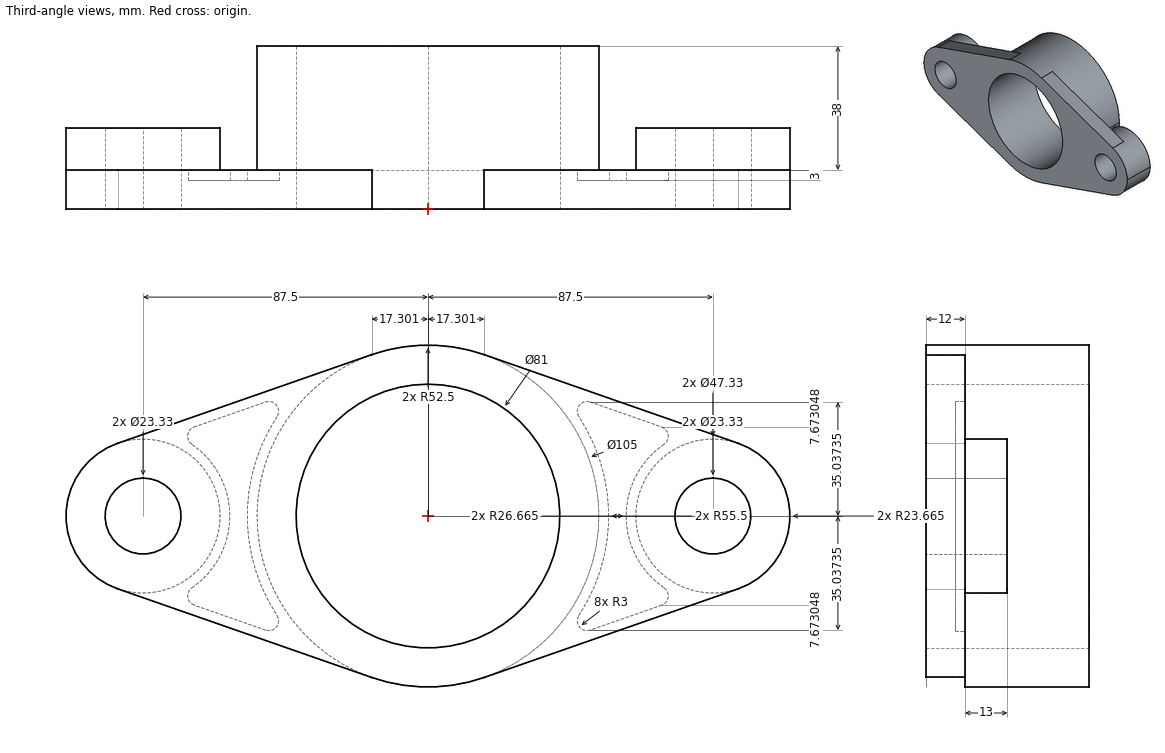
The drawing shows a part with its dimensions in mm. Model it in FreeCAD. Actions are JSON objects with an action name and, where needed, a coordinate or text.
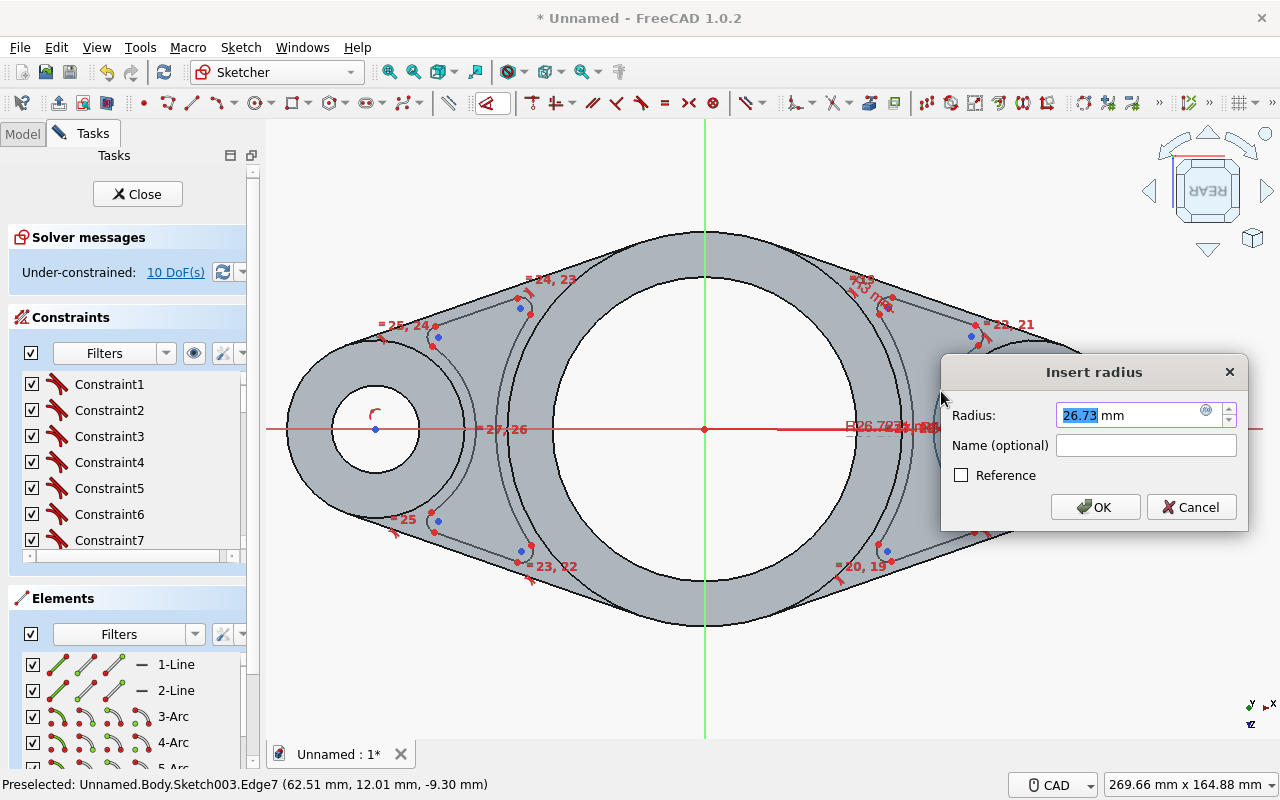
{"action": "type", "text": "26.665"}
{"action": "key", "text": "Return"}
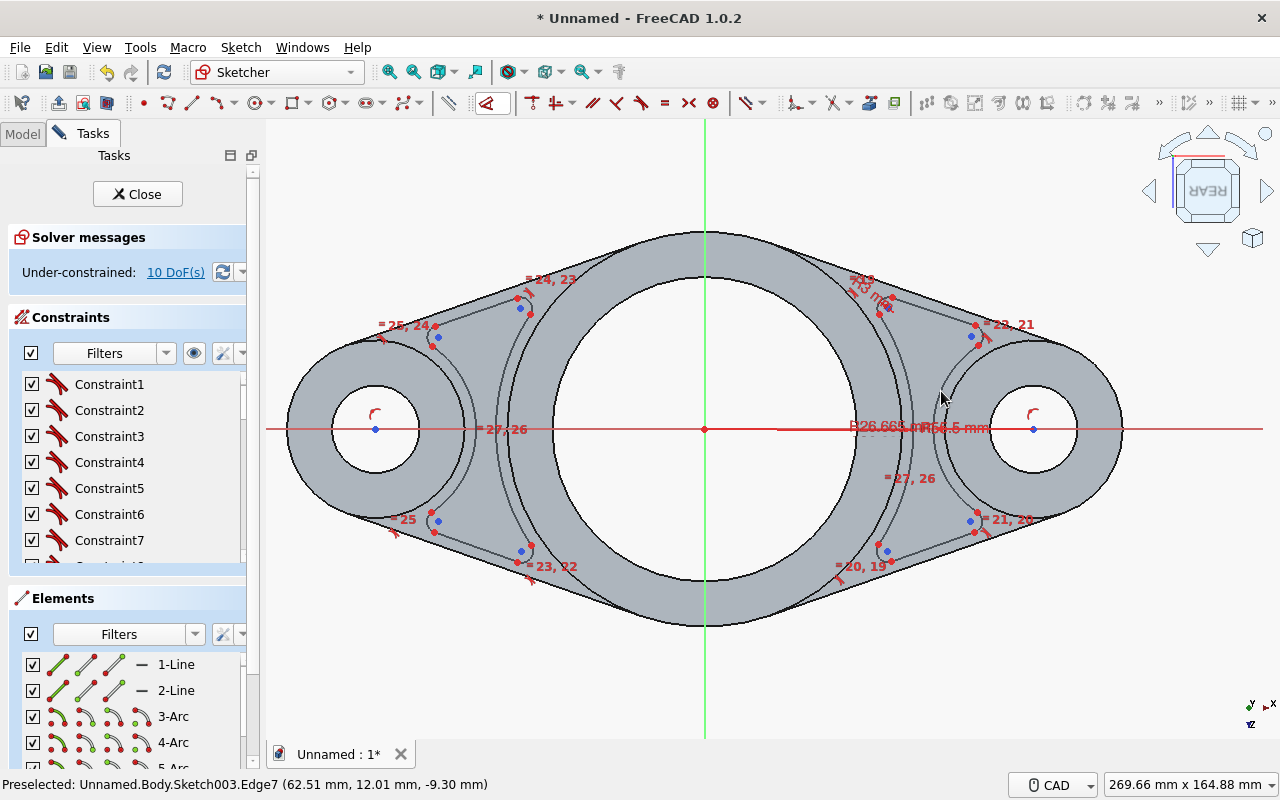
{"action": "left_click", "coordinate": [1034, 429]}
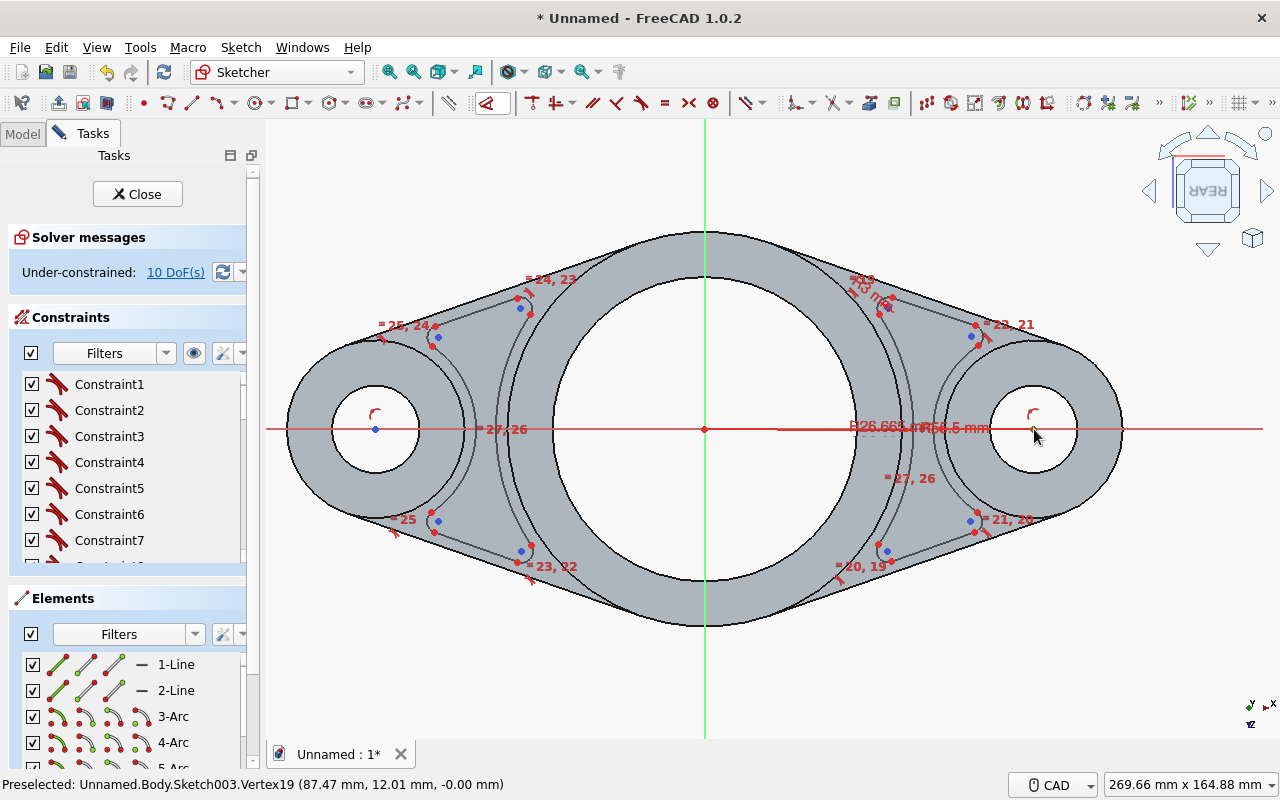
{"action": "left_click", "coordinate": [504, 104]}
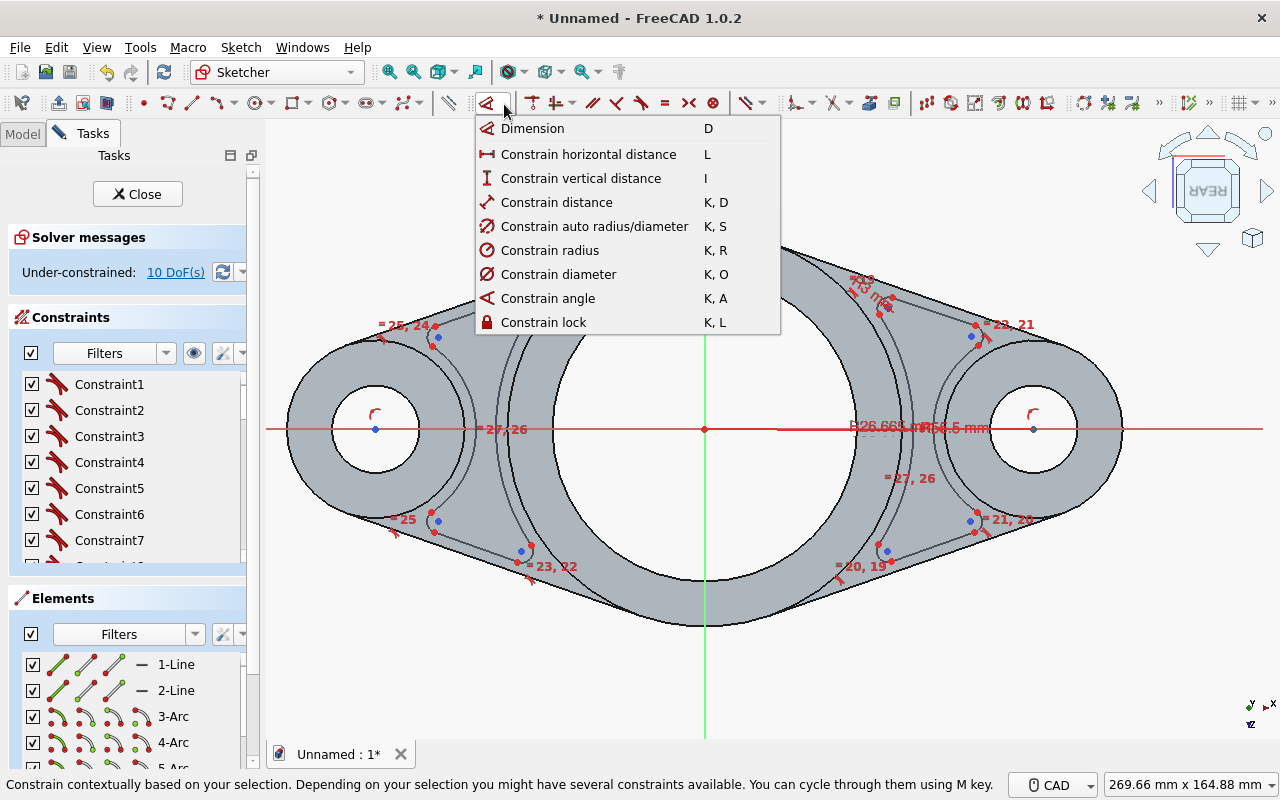
{"action": "left_click", "coordinate": [628, 154]}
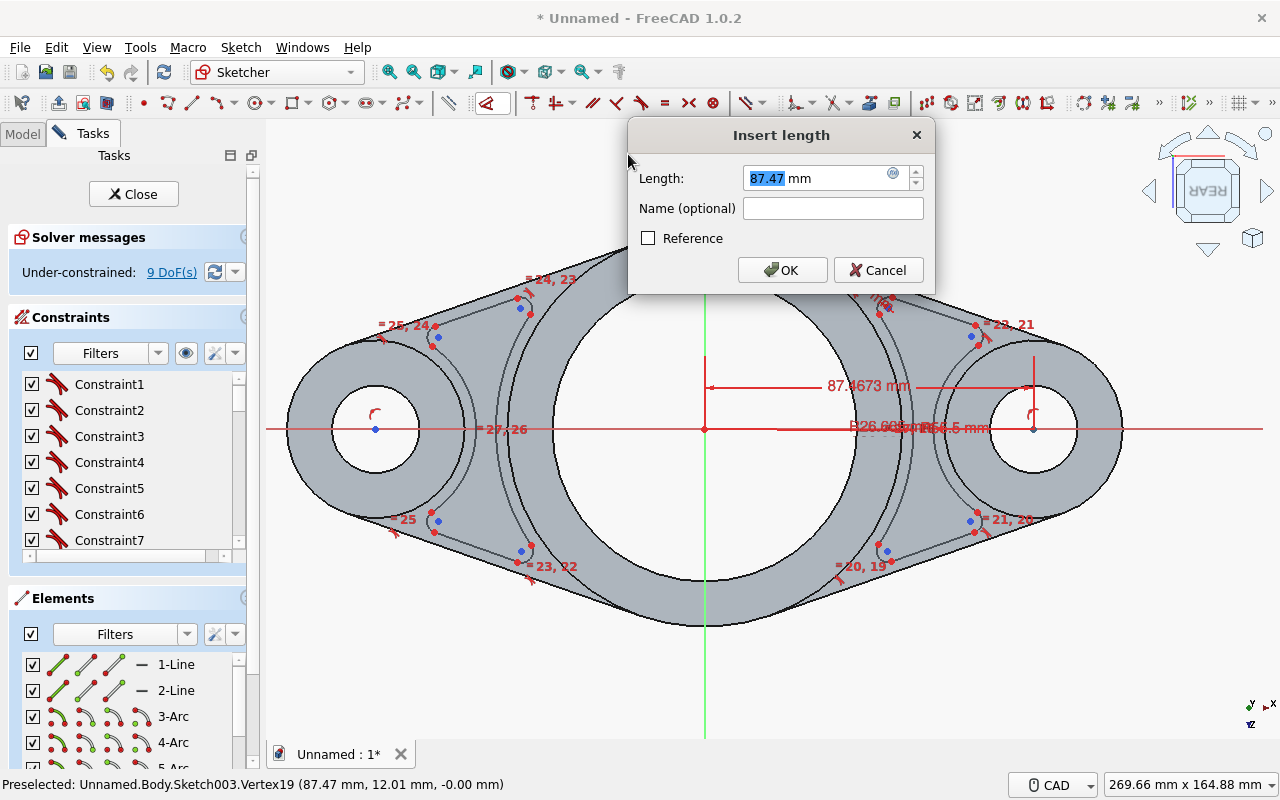
{"action": "type", "text": "87.5"}
{"action": "key", "text": "Return"}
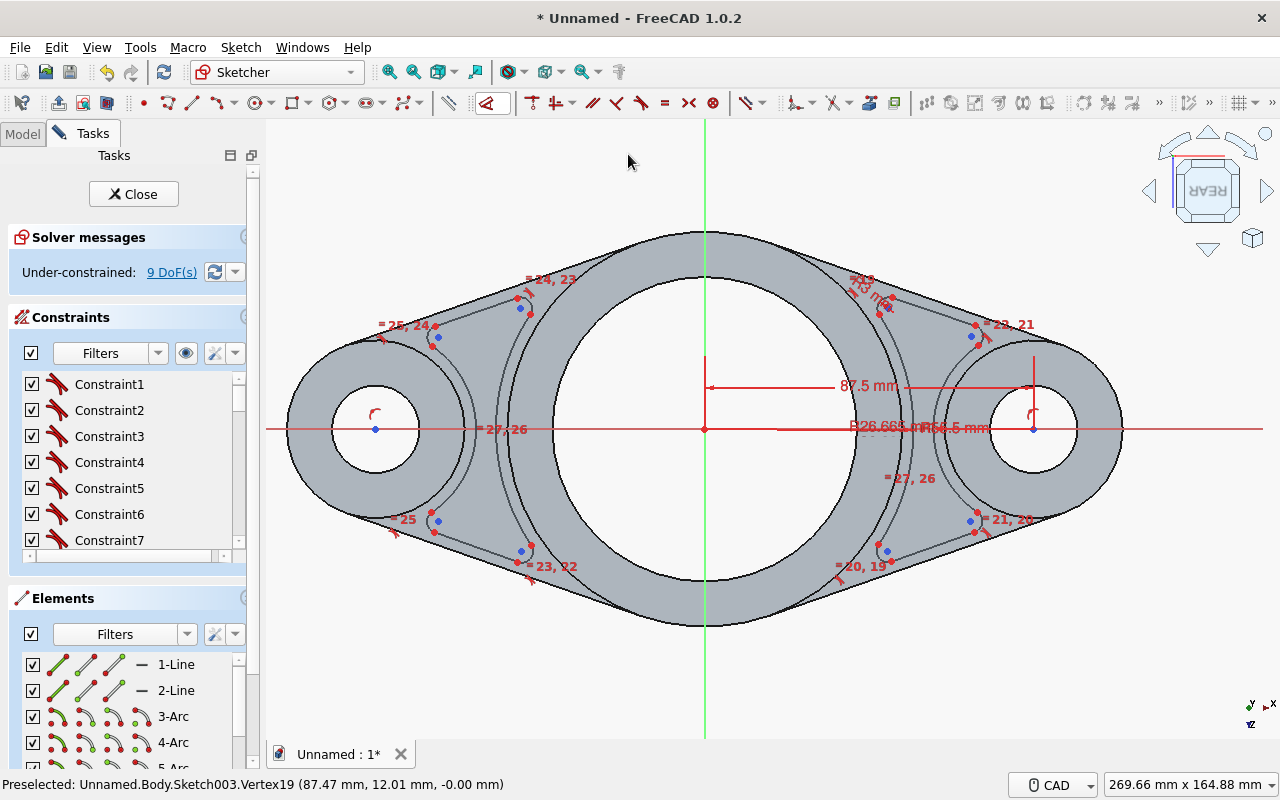
{"action": "left_click", "coordinate": [376, 429]}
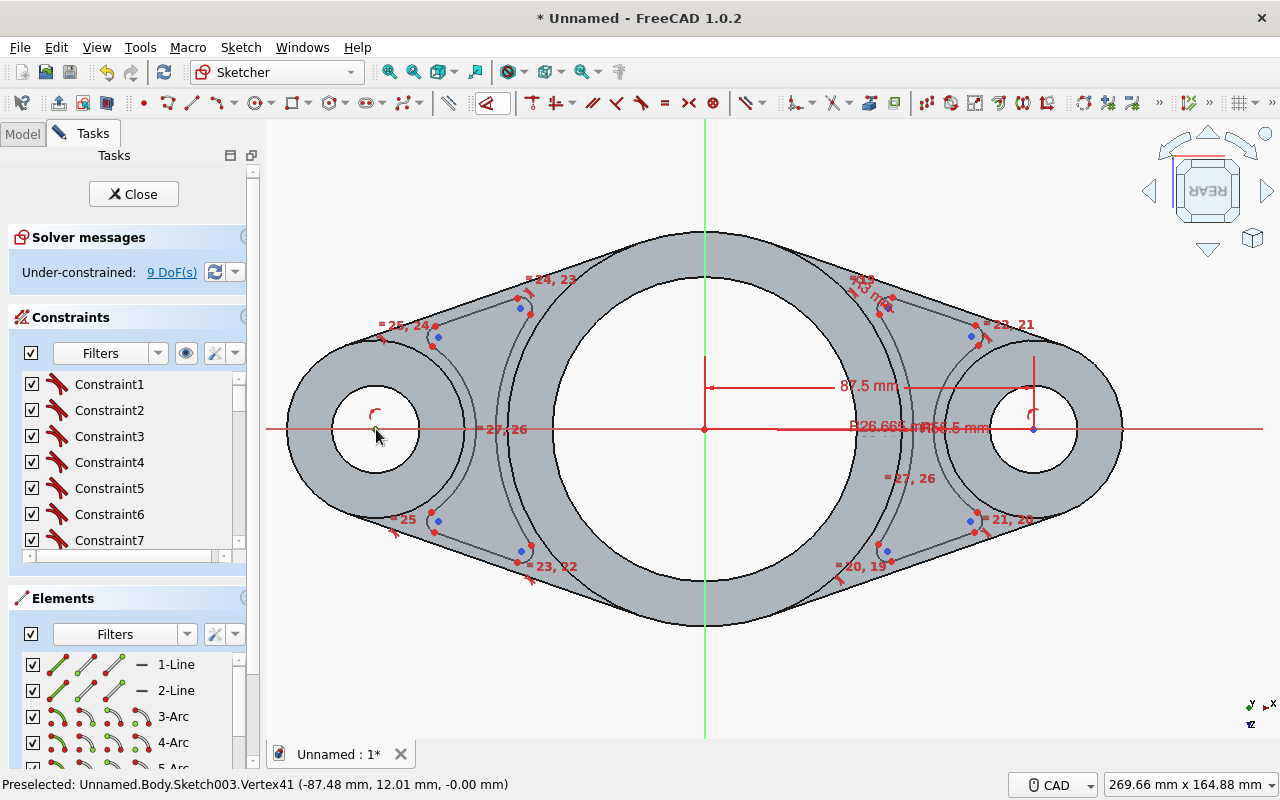
{"action": "left_click", "coordinate": [504, 104]}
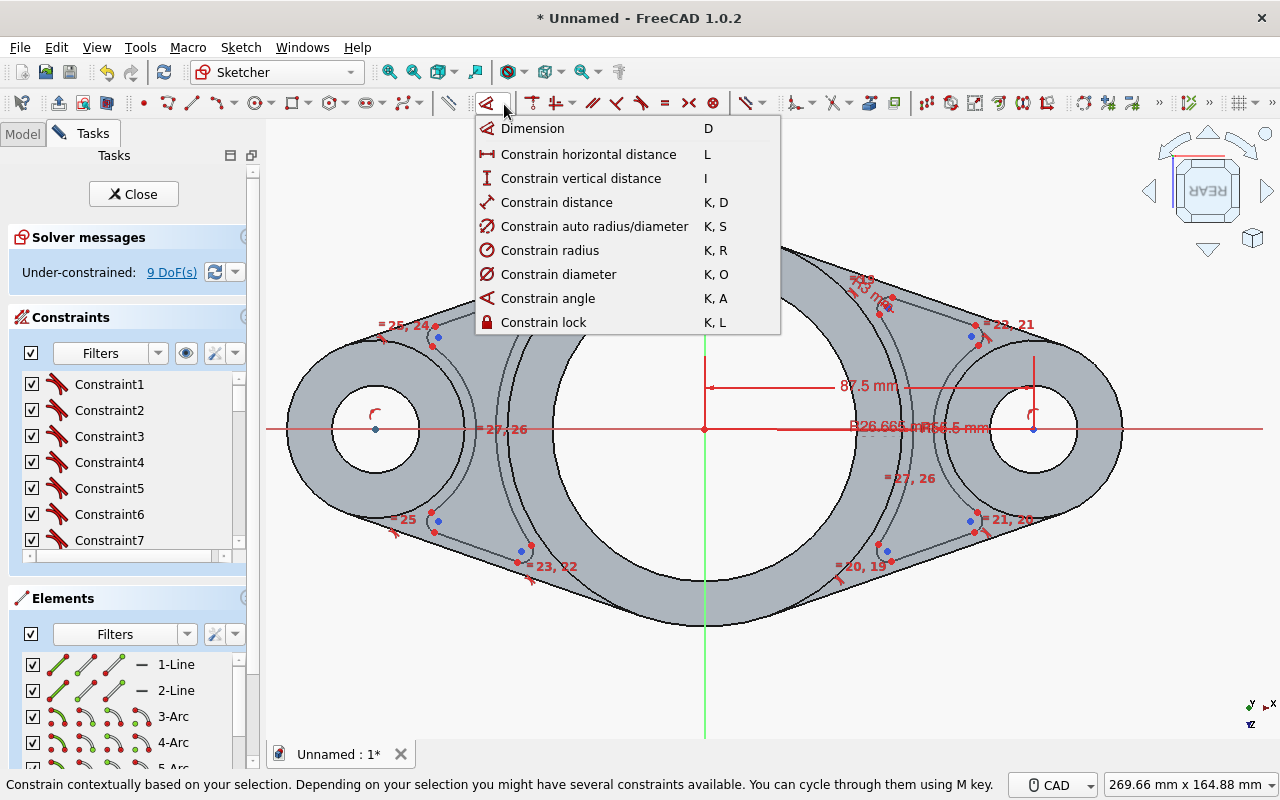
{"action": "left_click", "coordinate": [628, 154]}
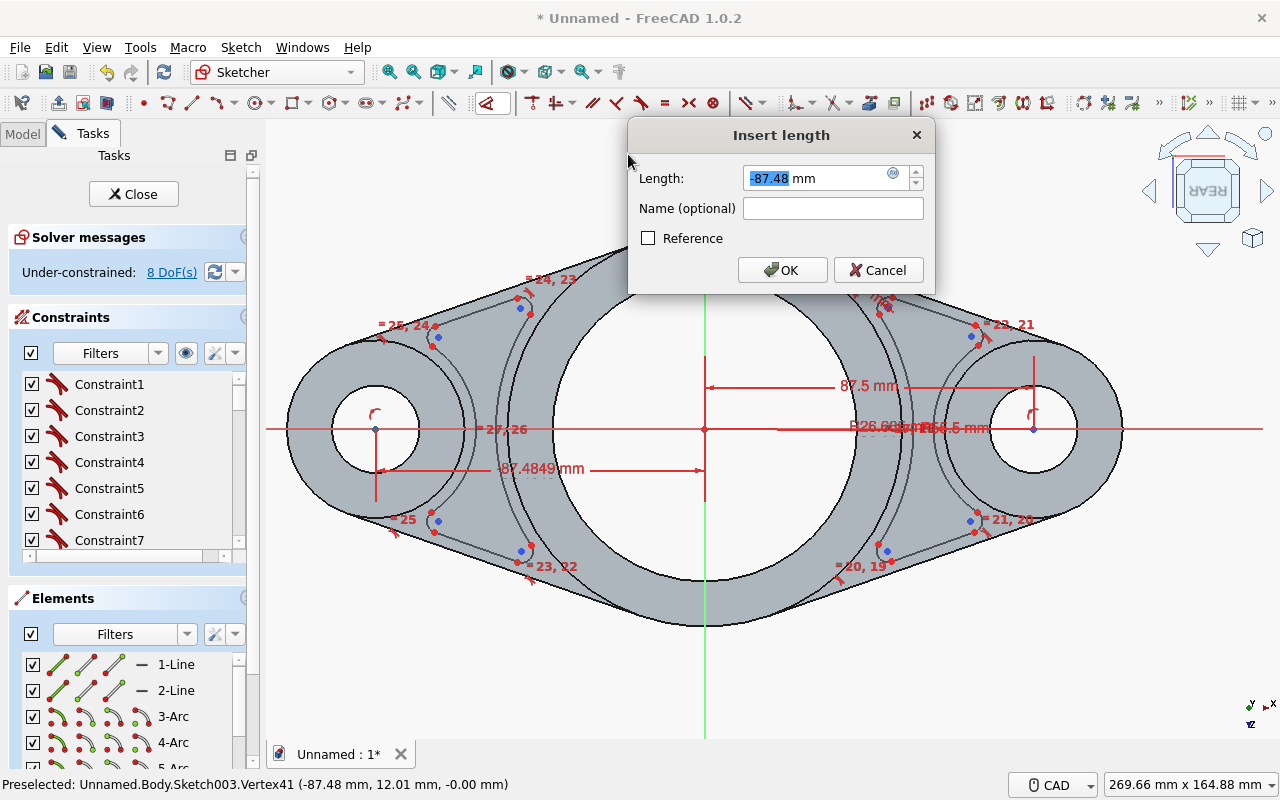
{"action": "type", "text": "-87.5"}
{"action": "key", "text": "Return"}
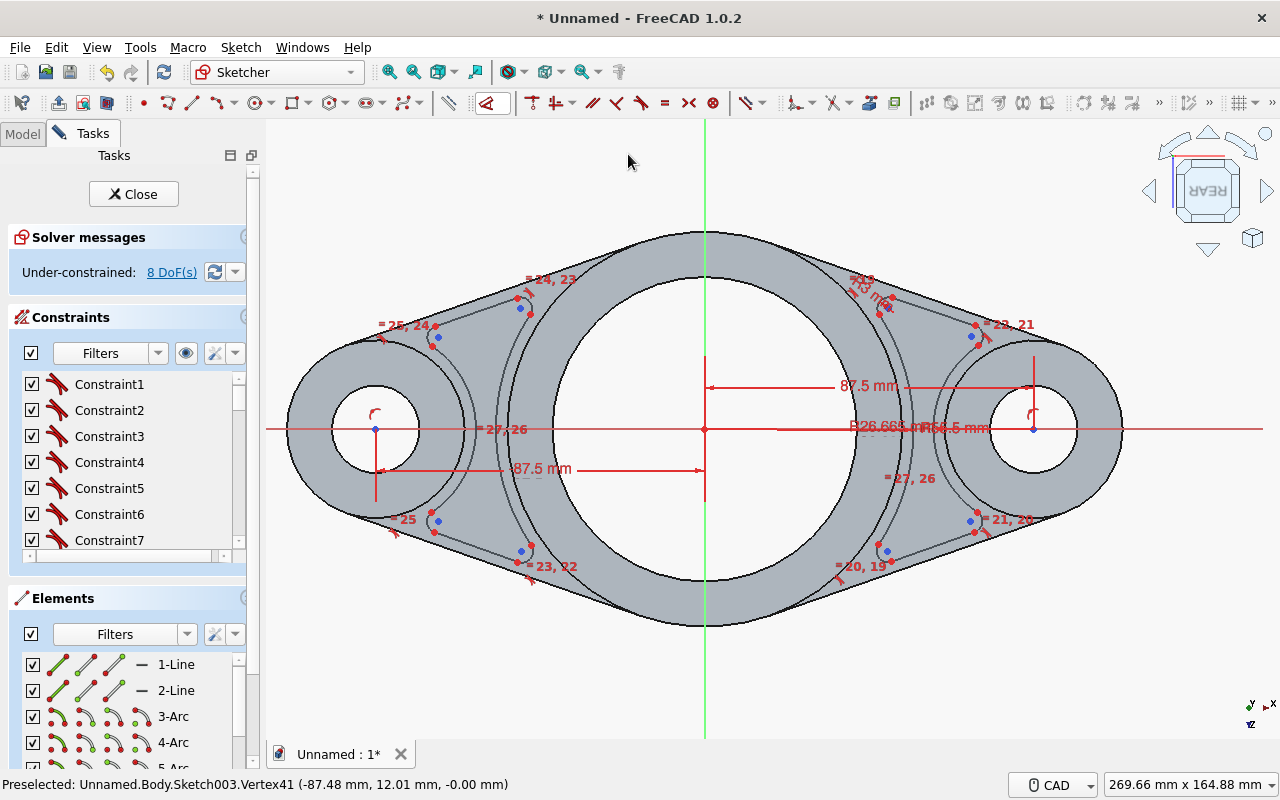
{"action": "left_click", "coordinate": [892, 298]}